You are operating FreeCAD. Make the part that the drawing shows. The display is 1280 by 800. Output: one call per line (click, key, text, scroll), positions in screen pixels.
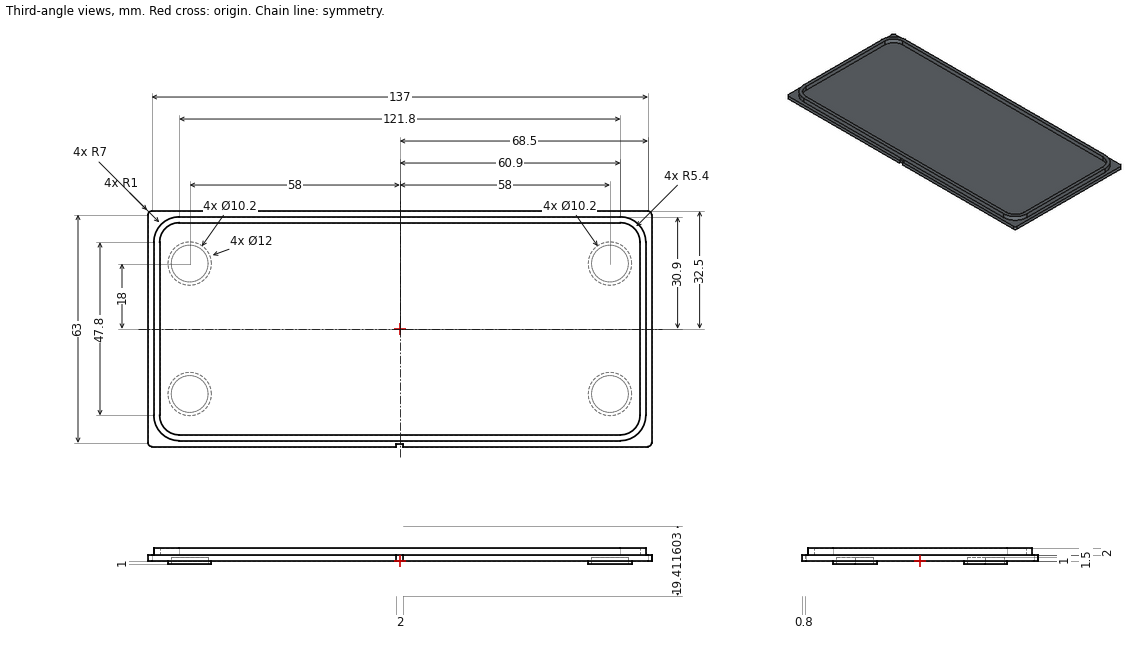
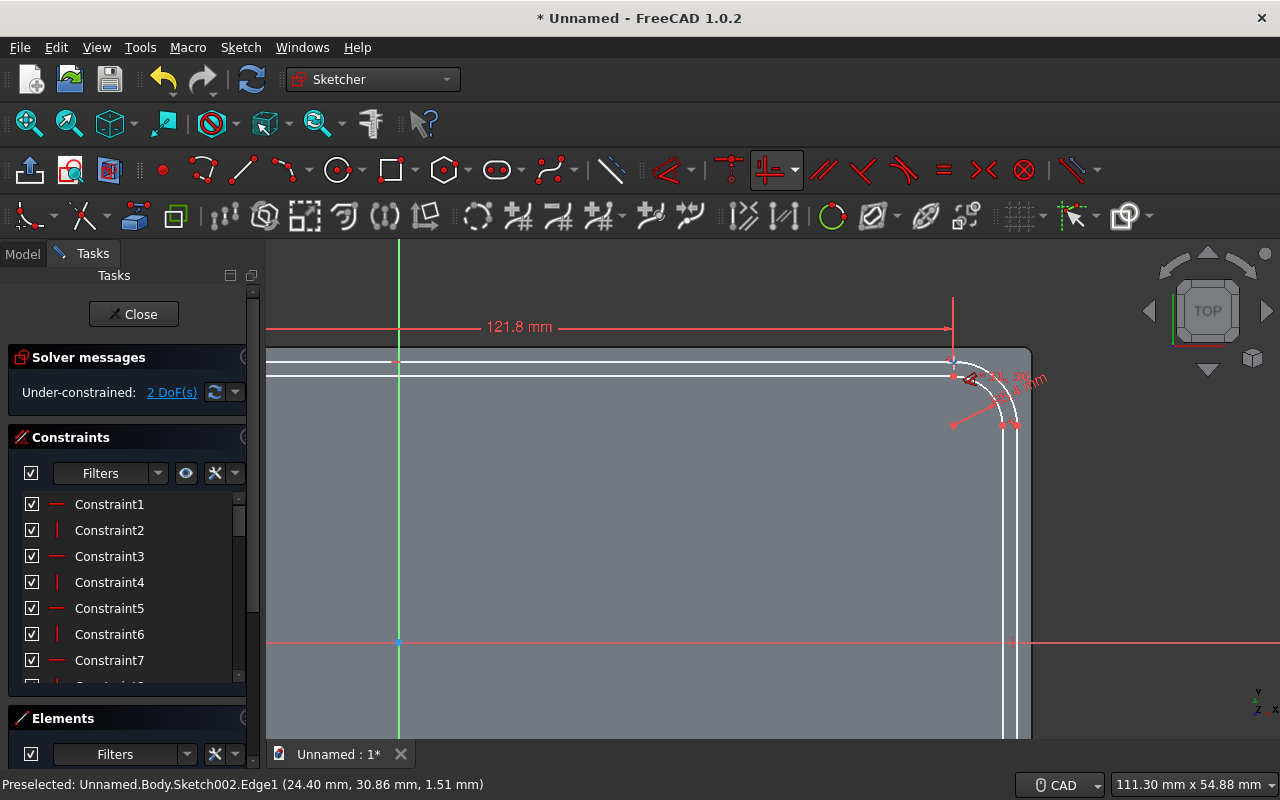
click(953, 362)
click(676, 328)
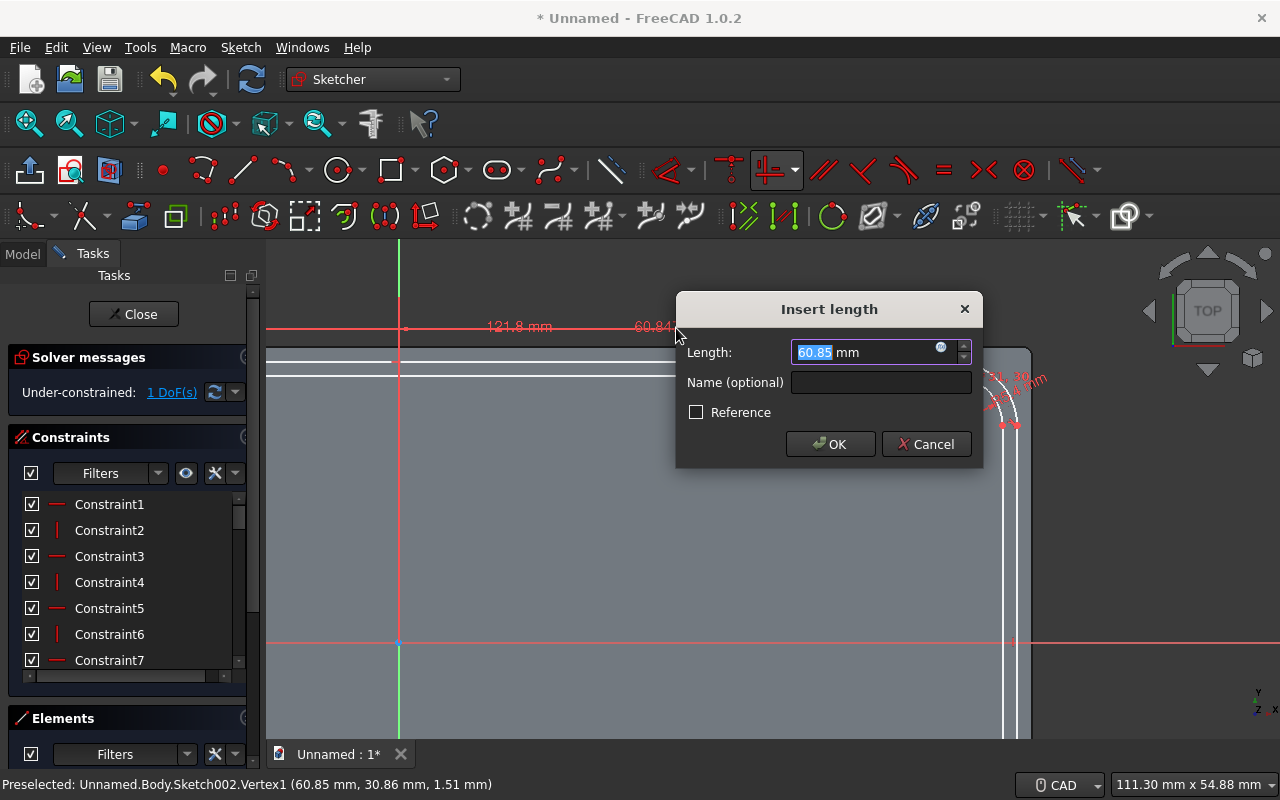
text(60.9)
key(Return)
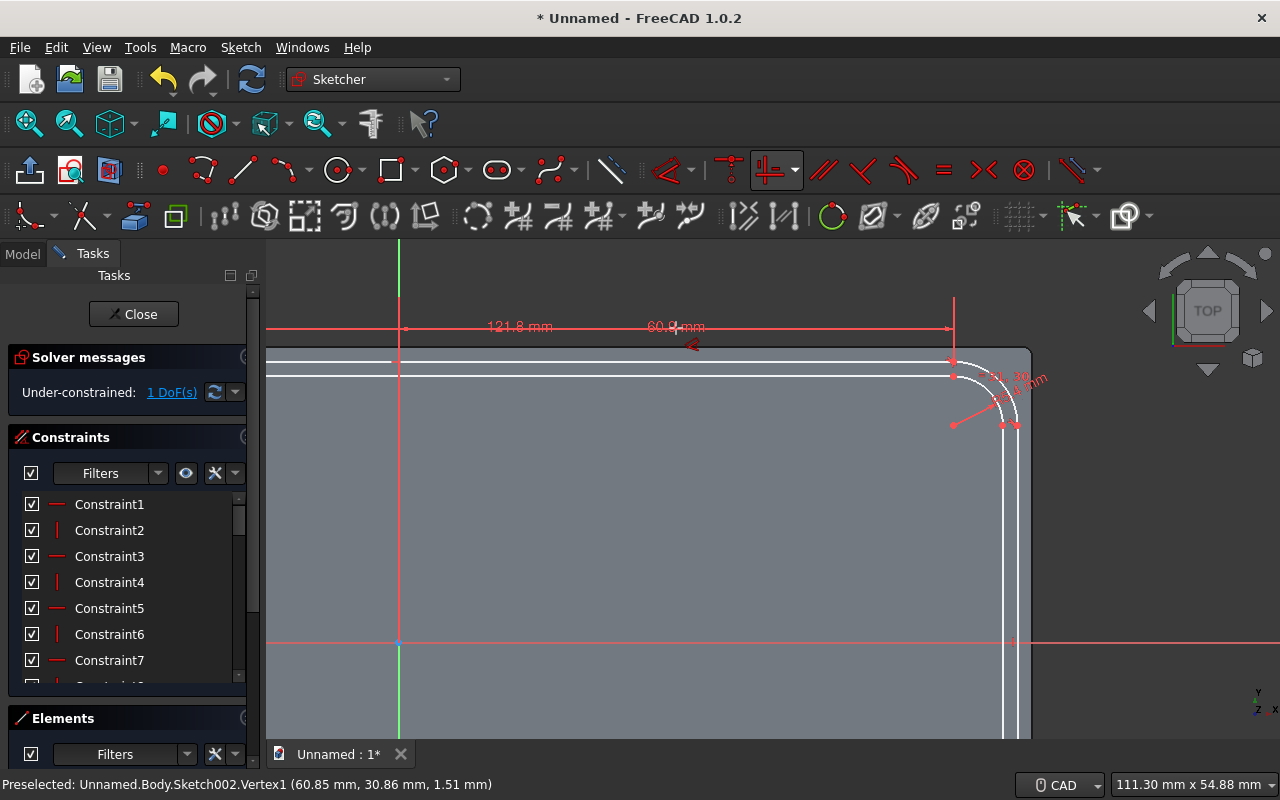
click(954, 362)
click(988, 502)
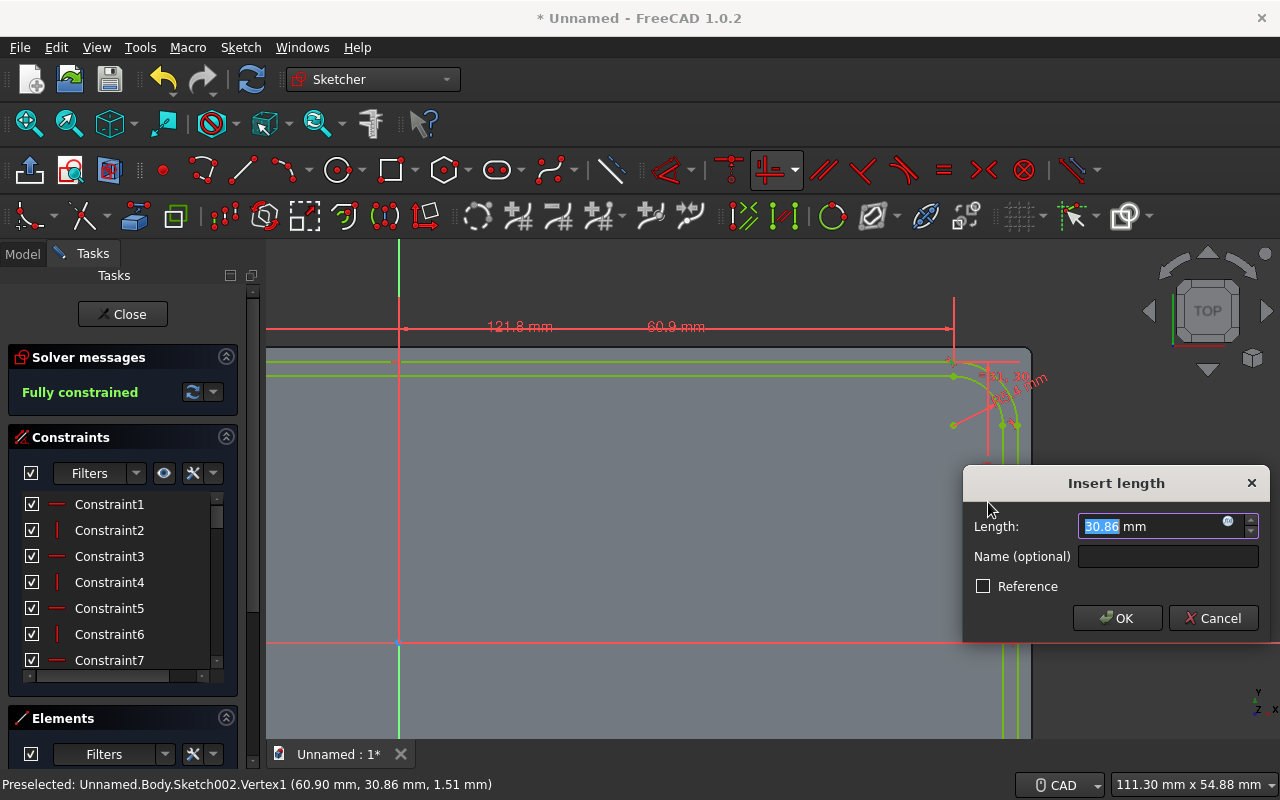
text(30.9)
key(Return)
key(Escape)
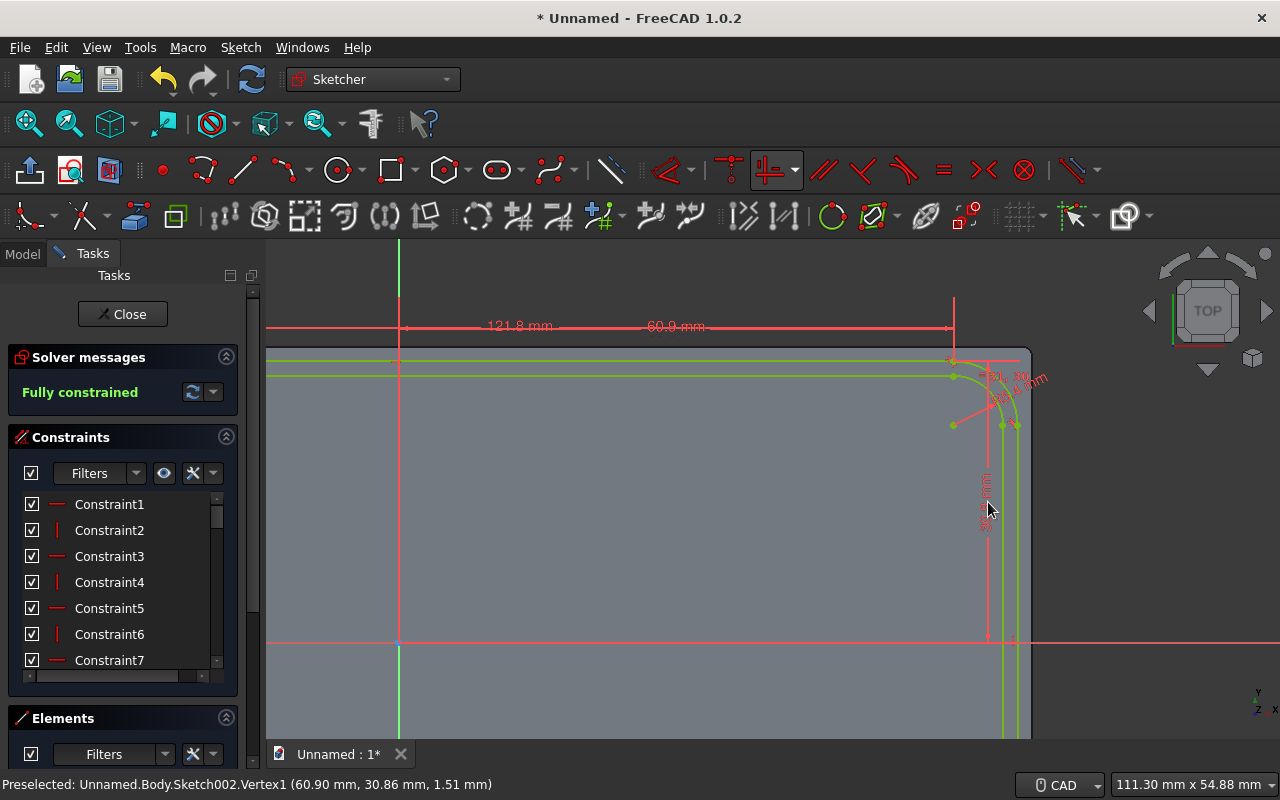
click(123, 314)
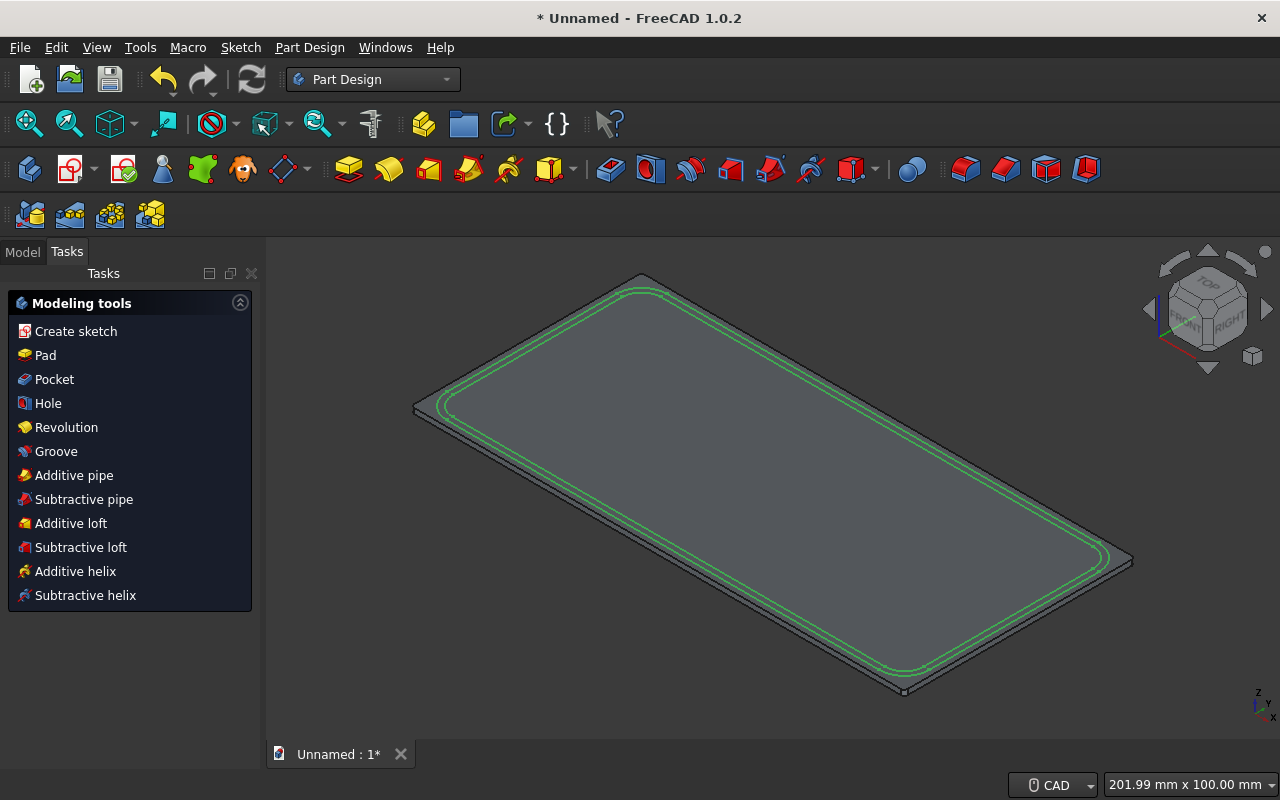
click(350, 170)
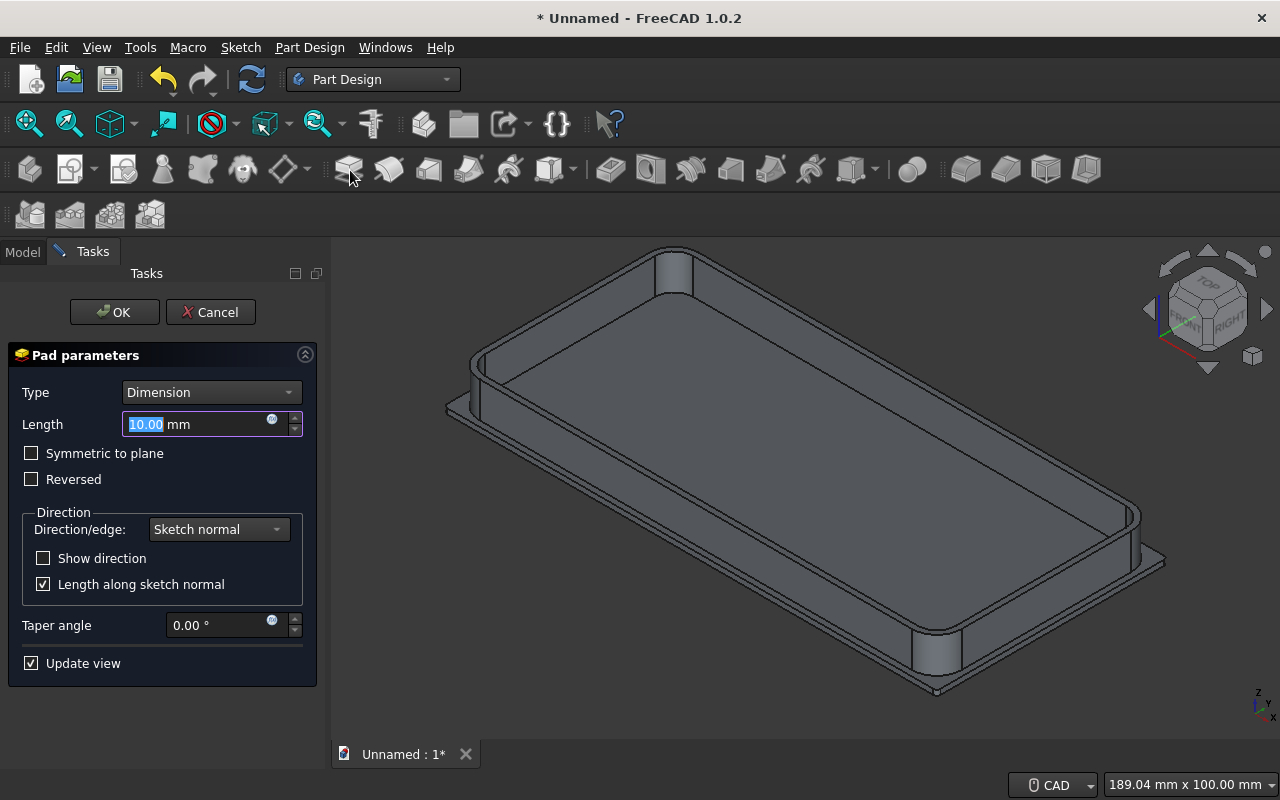
text(2)
key(Tab)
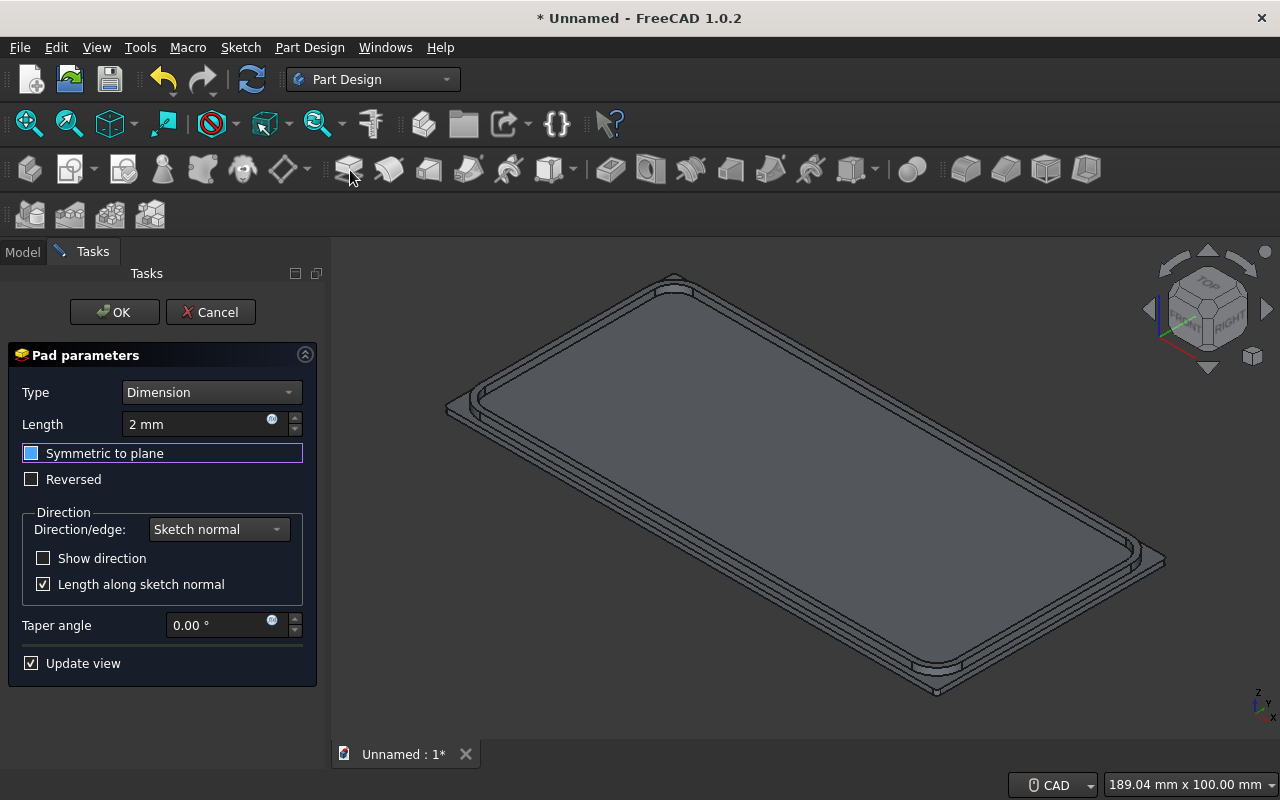
click(115, 312)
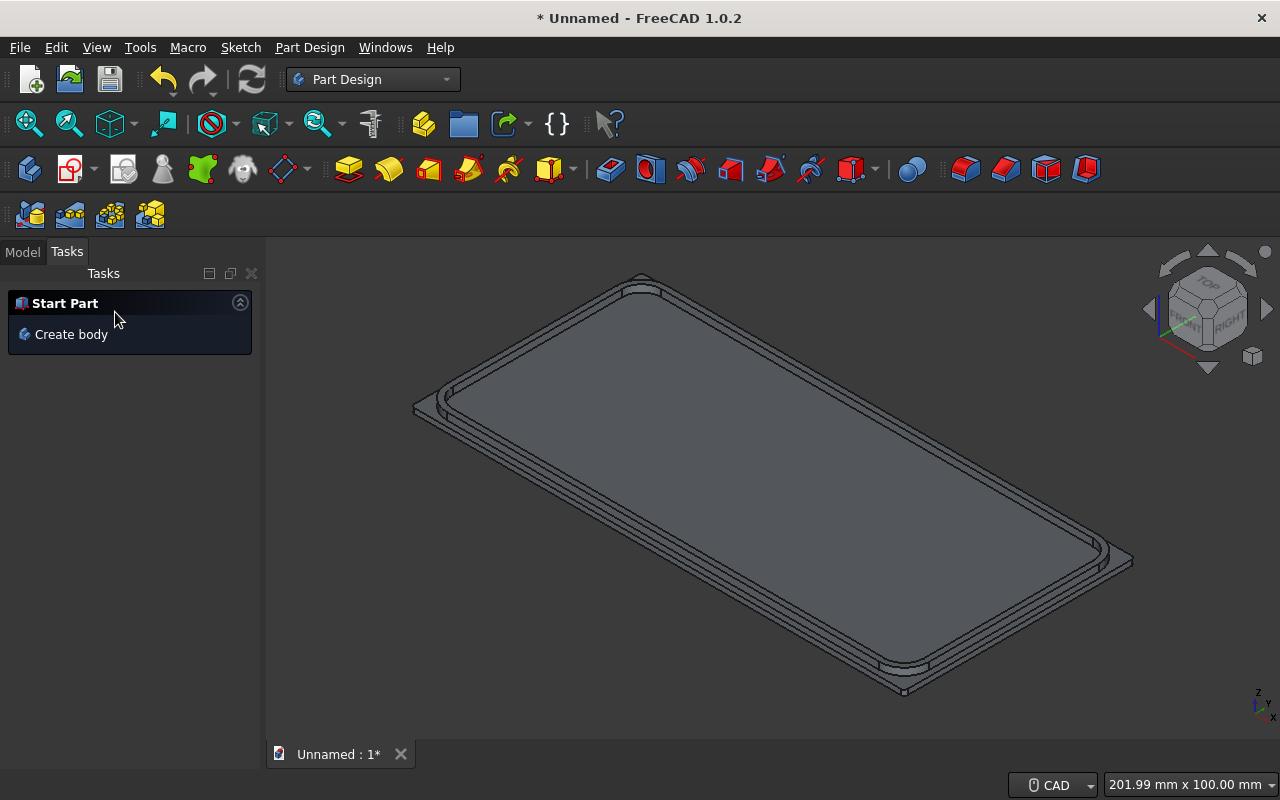
scroll(866, 671, up, 6)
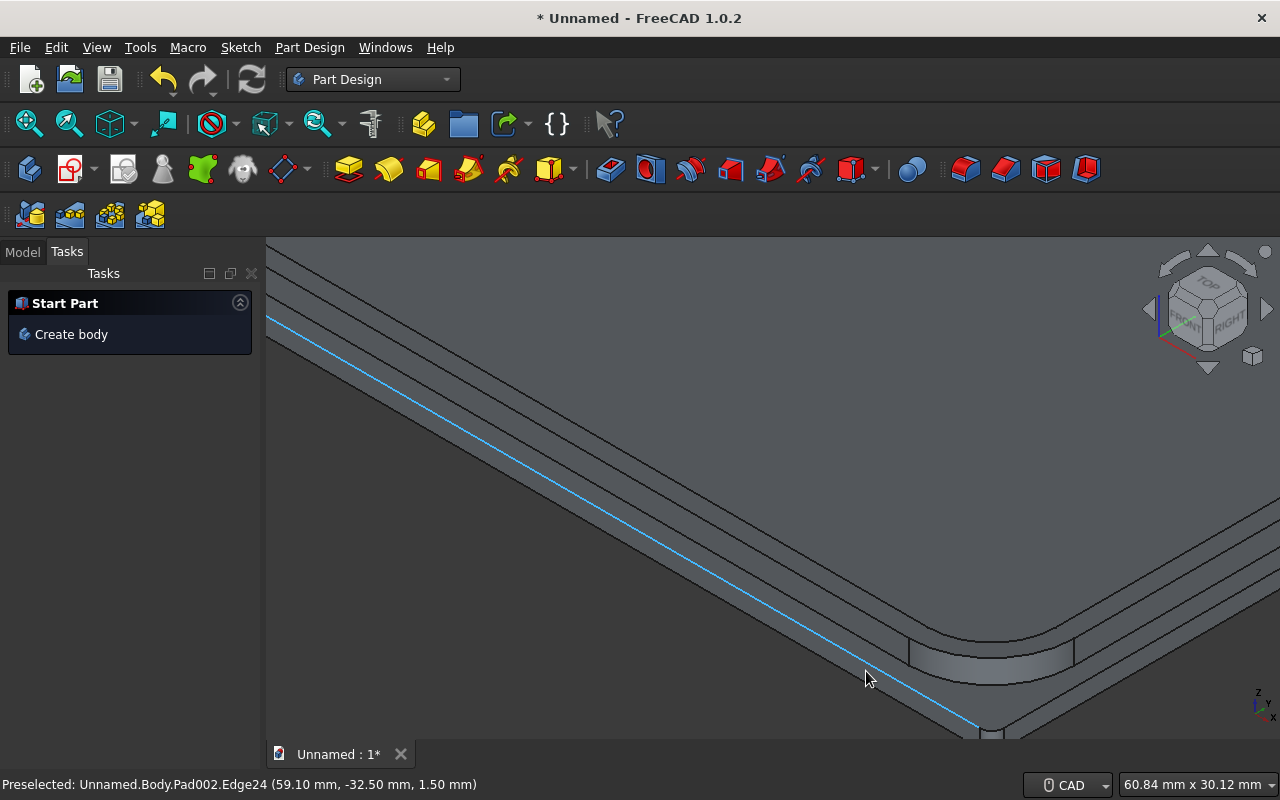
click(634, 538)